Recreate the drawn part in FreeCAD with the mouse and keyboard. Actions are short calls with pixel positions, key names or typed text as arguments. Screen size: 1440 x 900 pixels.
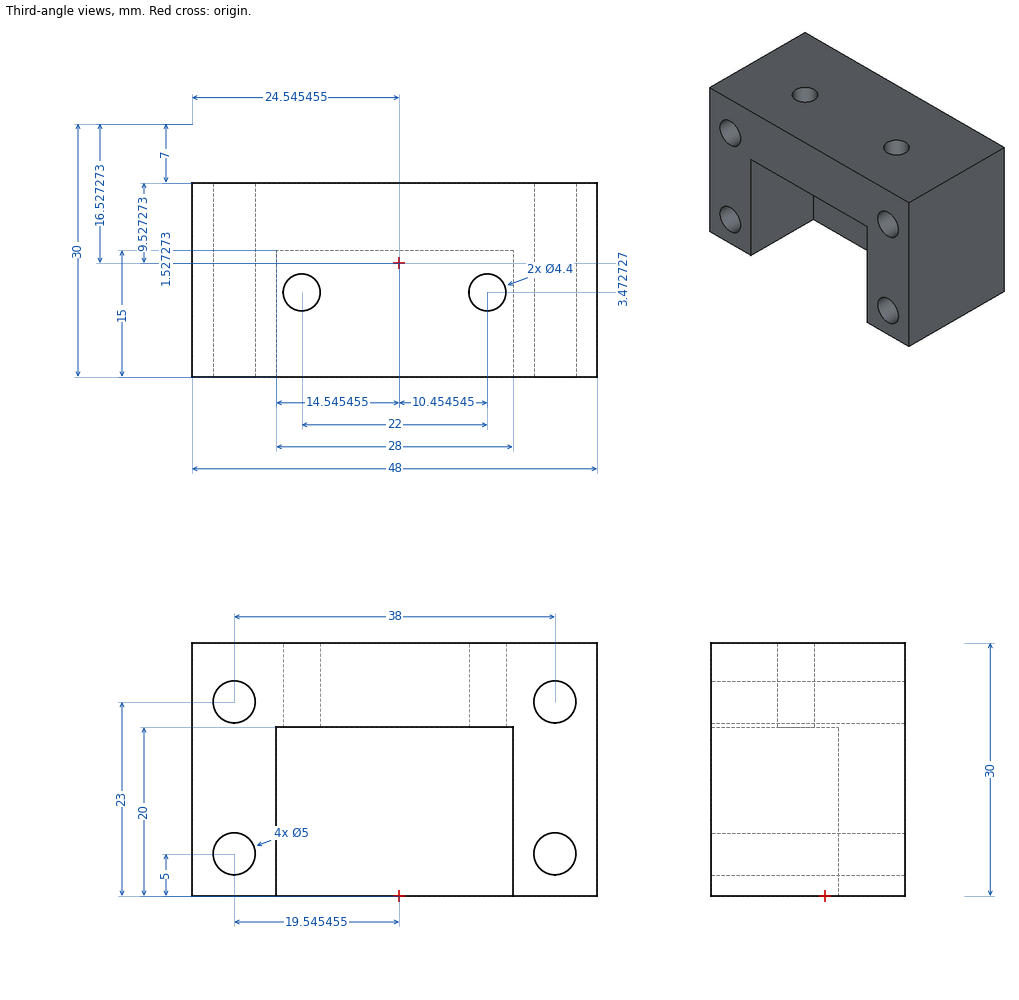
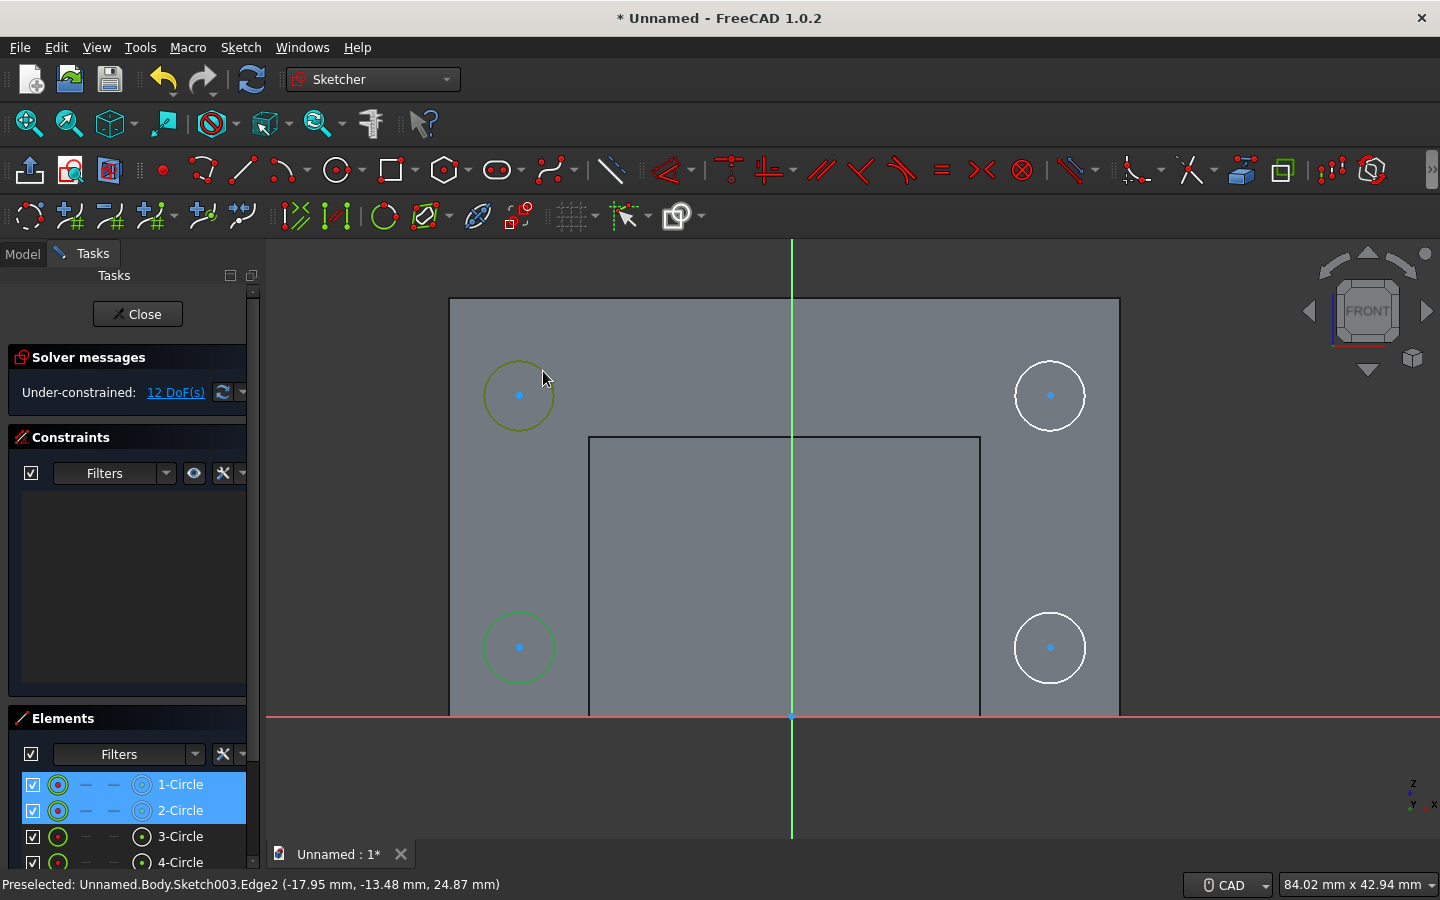
click(1074, 371)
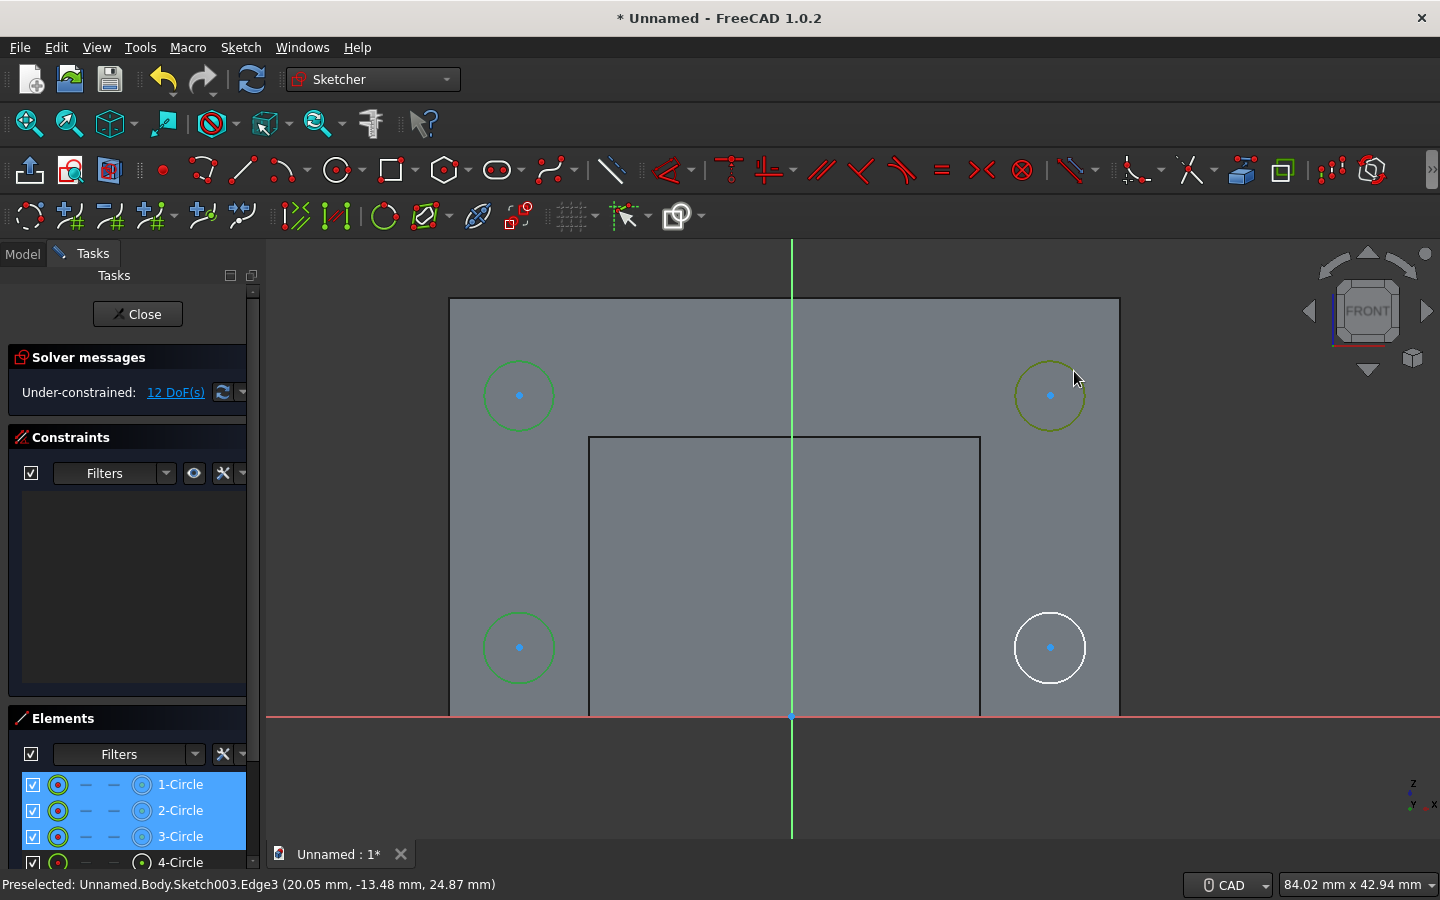
click(1075, 623)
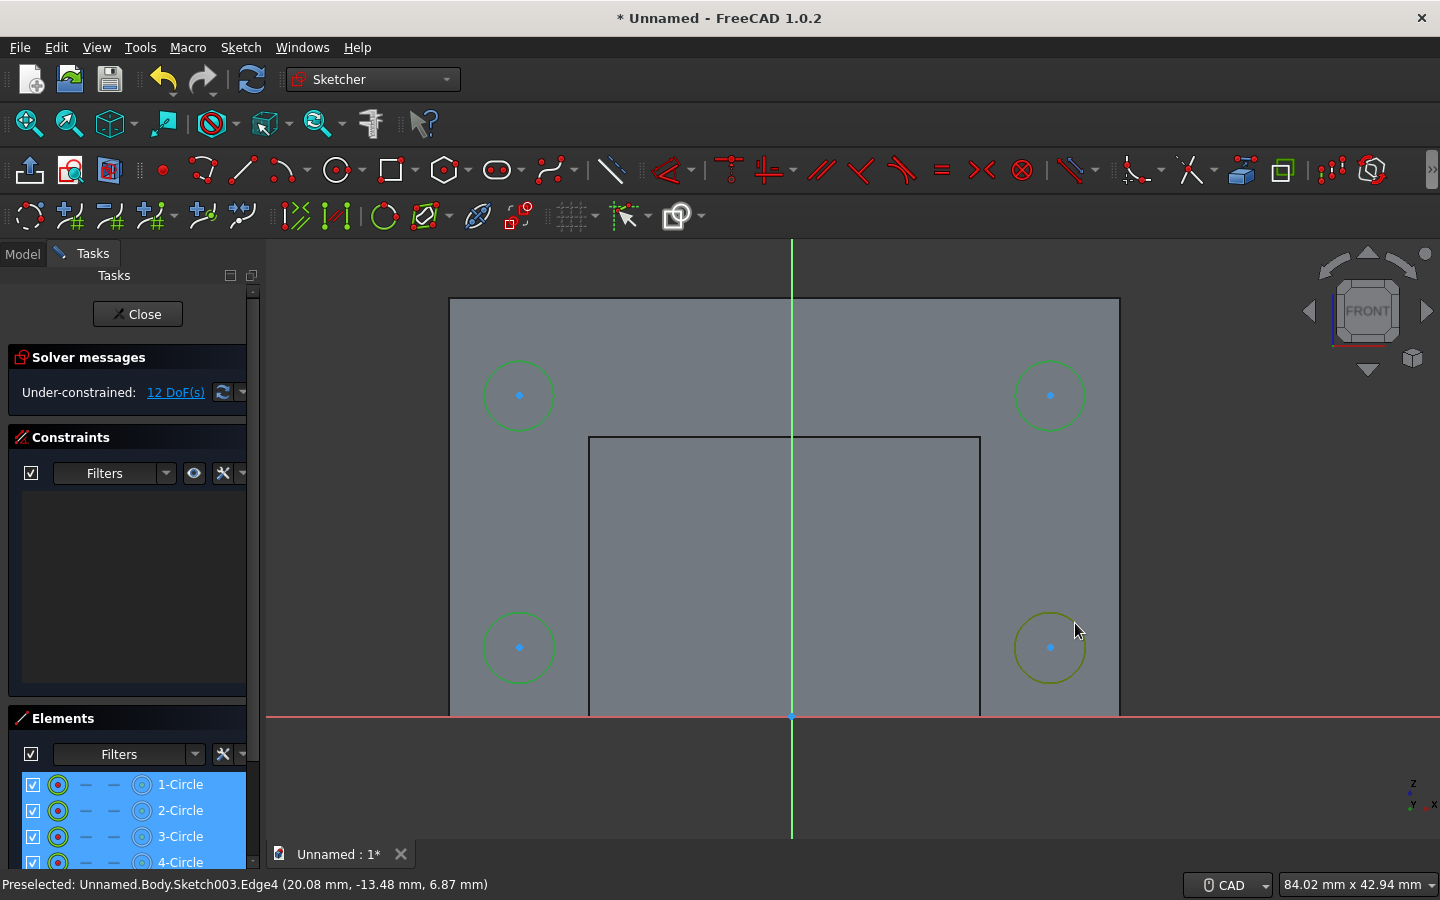
click(942, 170)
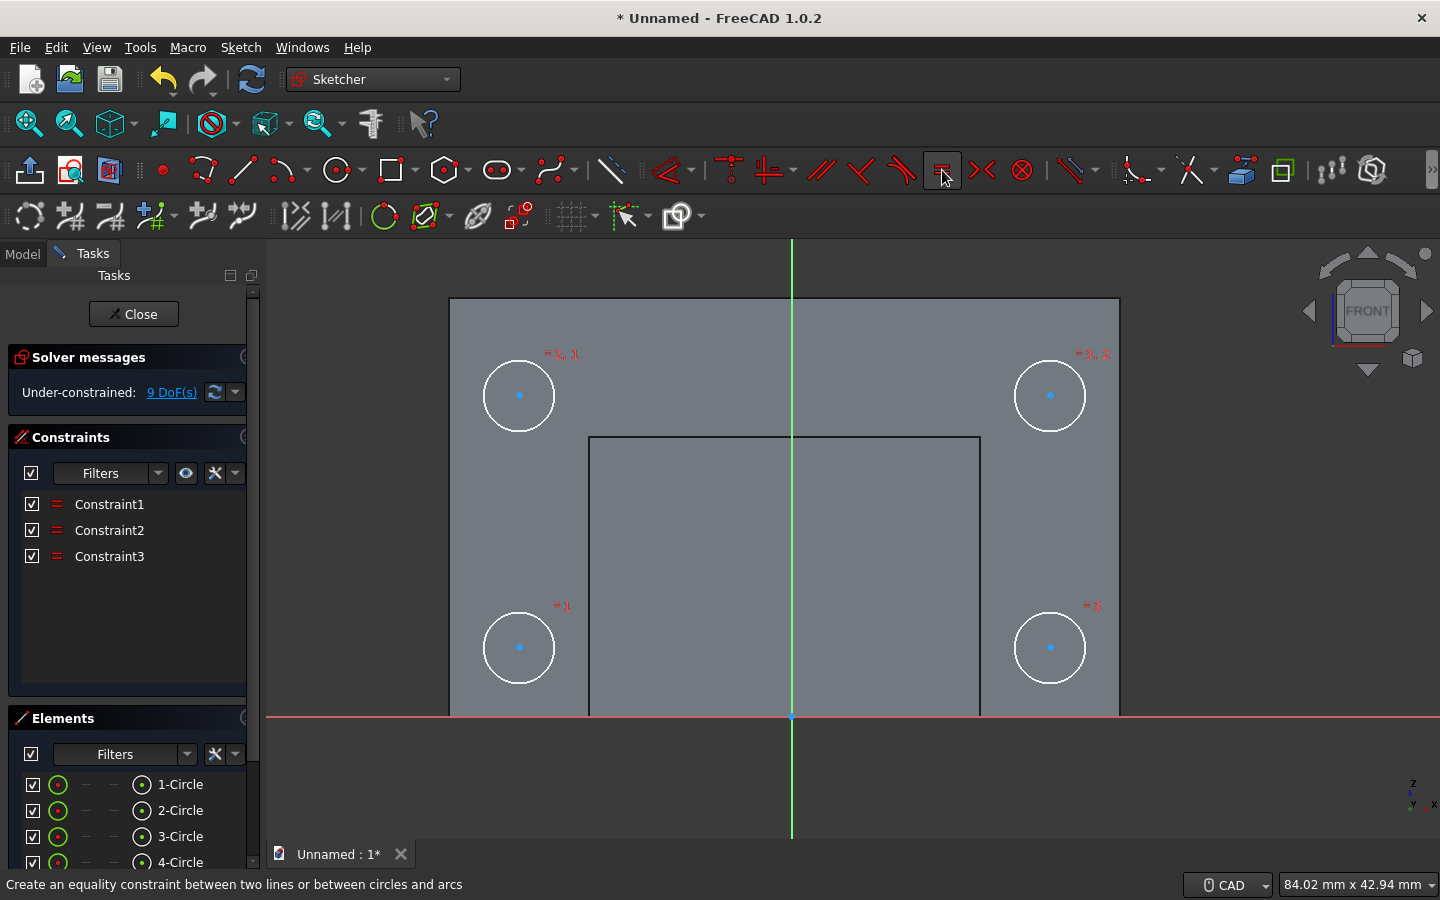
click(666, 170)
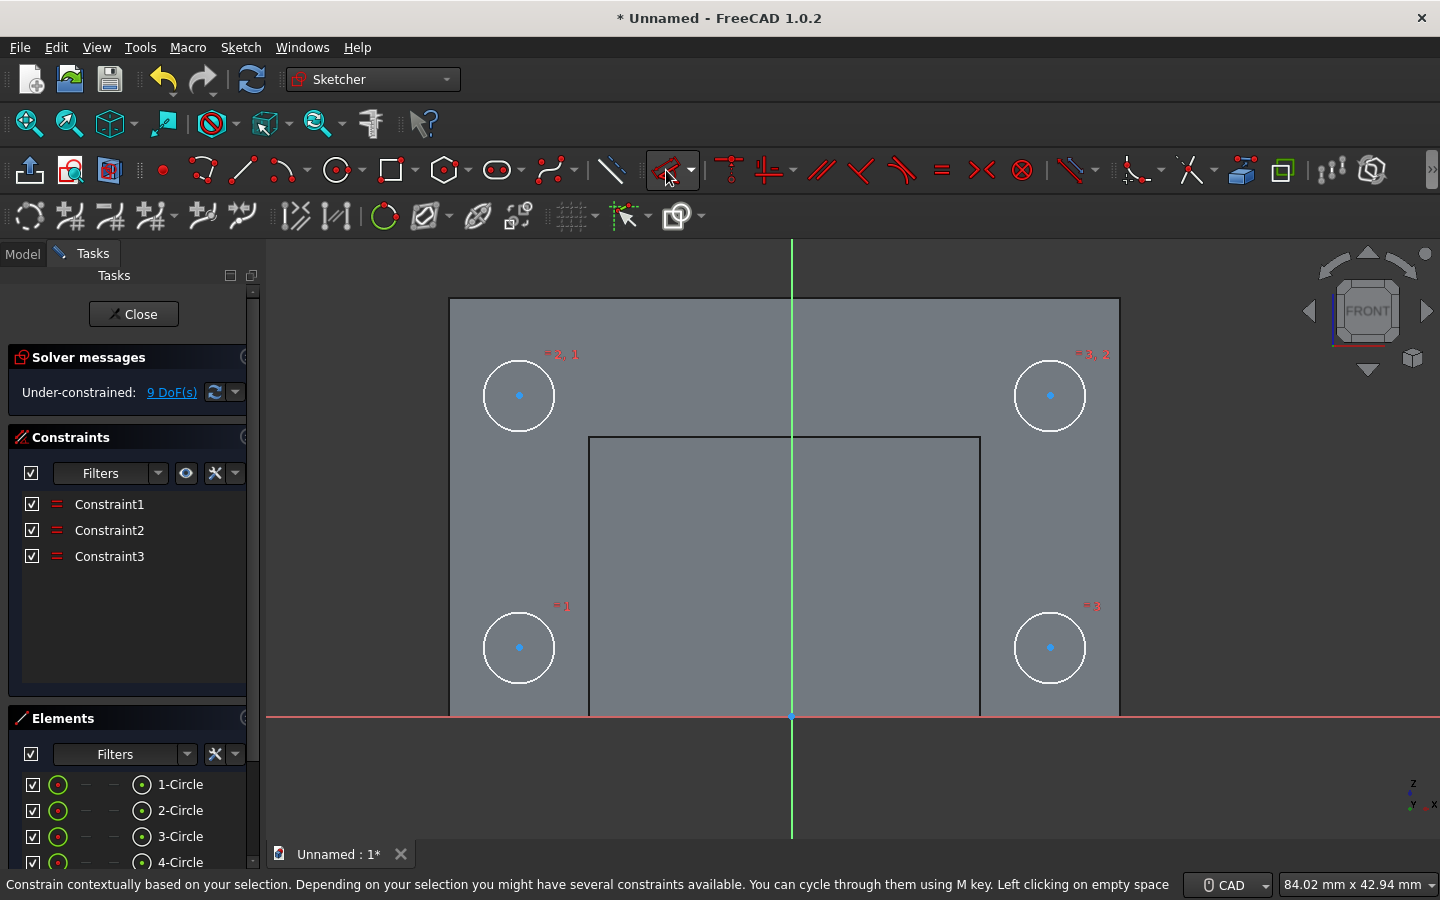
click(544, 623)
click(567, 600)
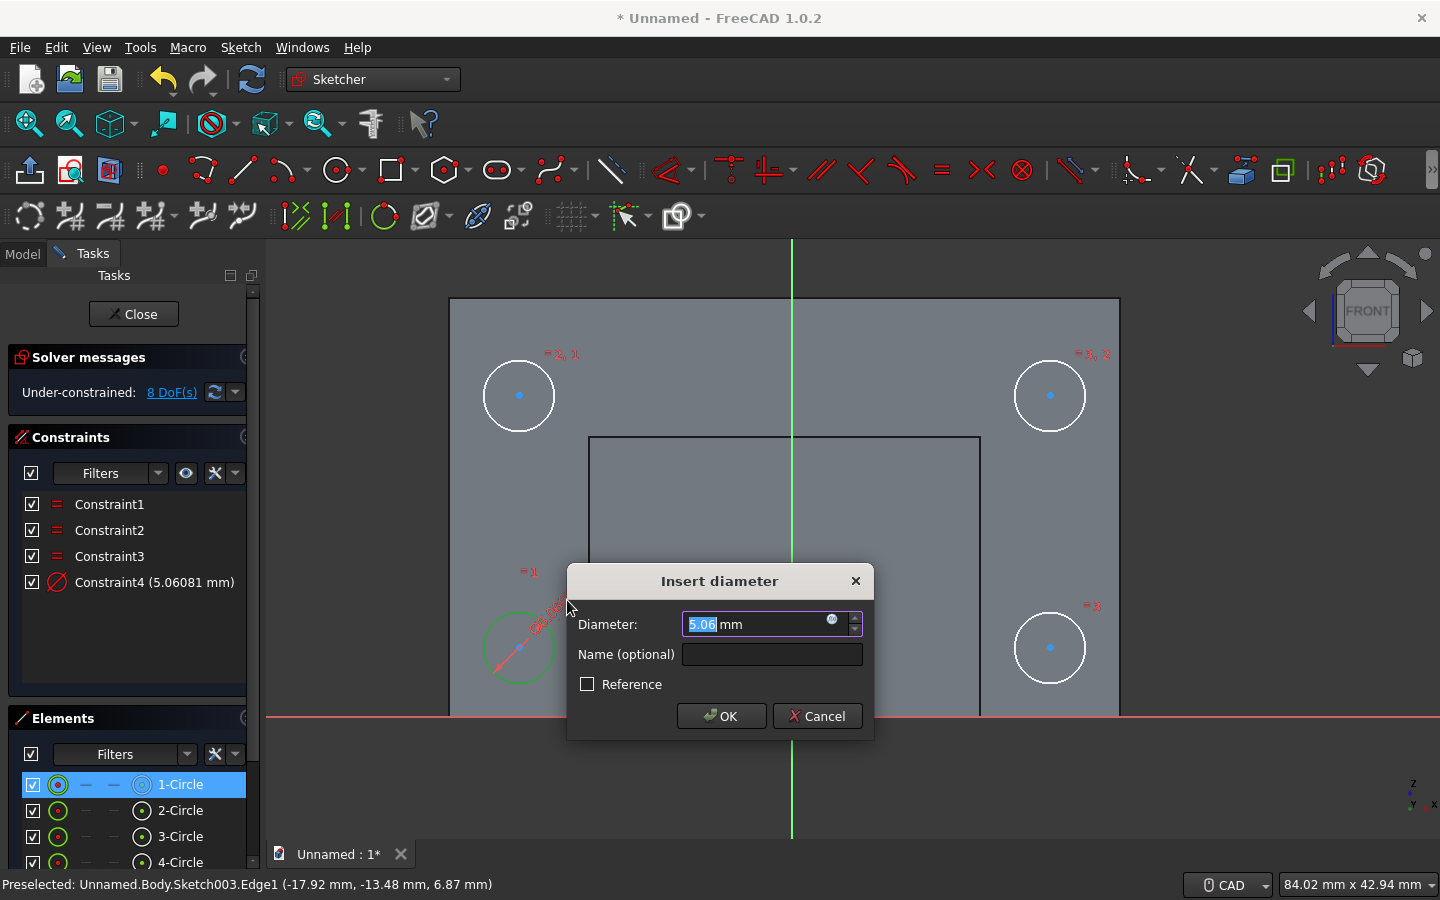
text(5)
key(Return)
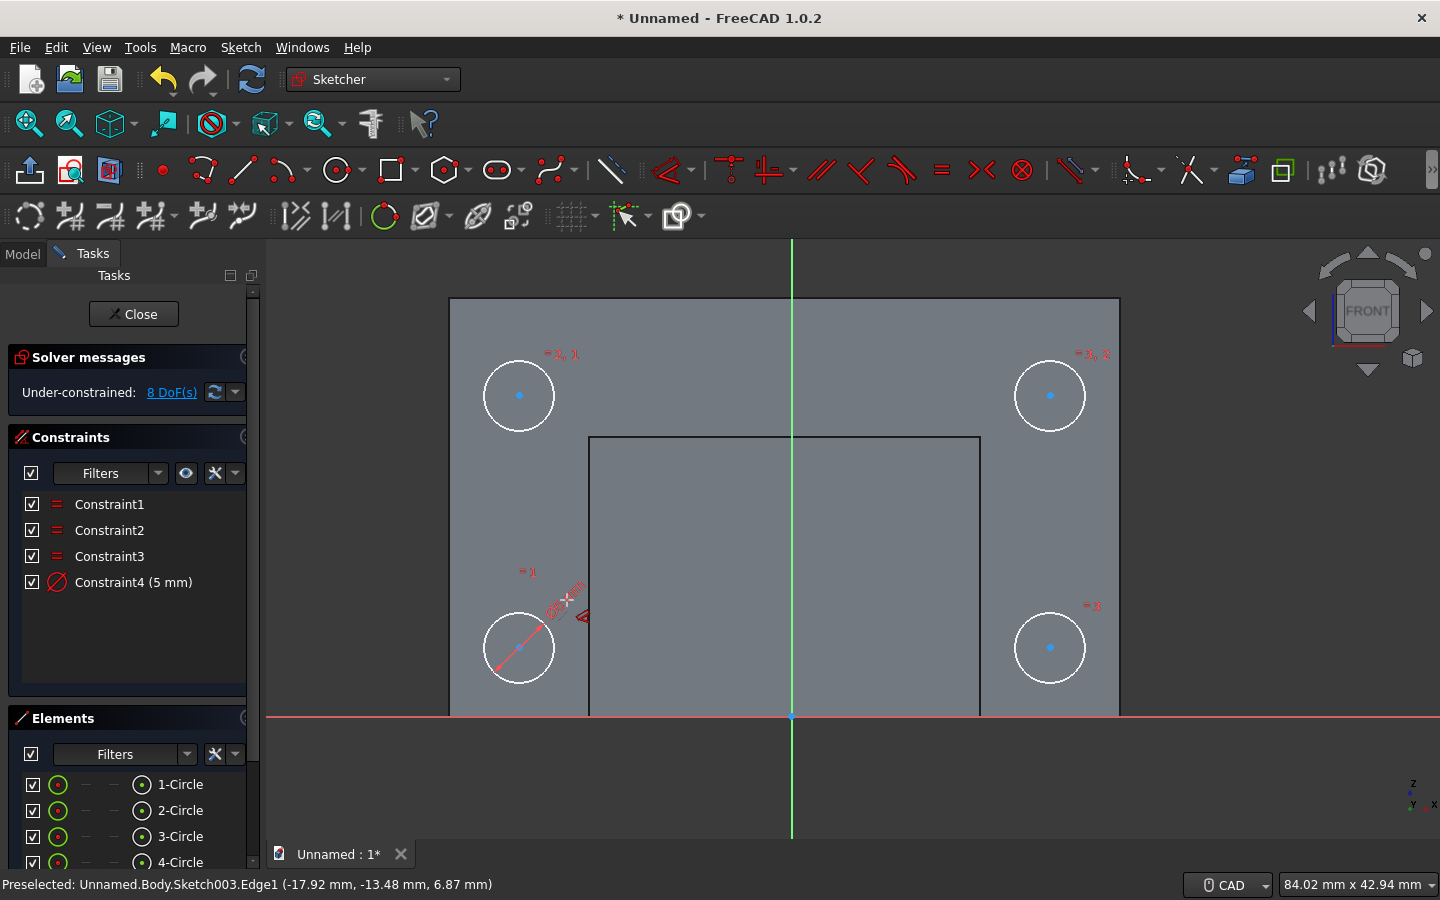
click(519, 648)
click(485, 682)